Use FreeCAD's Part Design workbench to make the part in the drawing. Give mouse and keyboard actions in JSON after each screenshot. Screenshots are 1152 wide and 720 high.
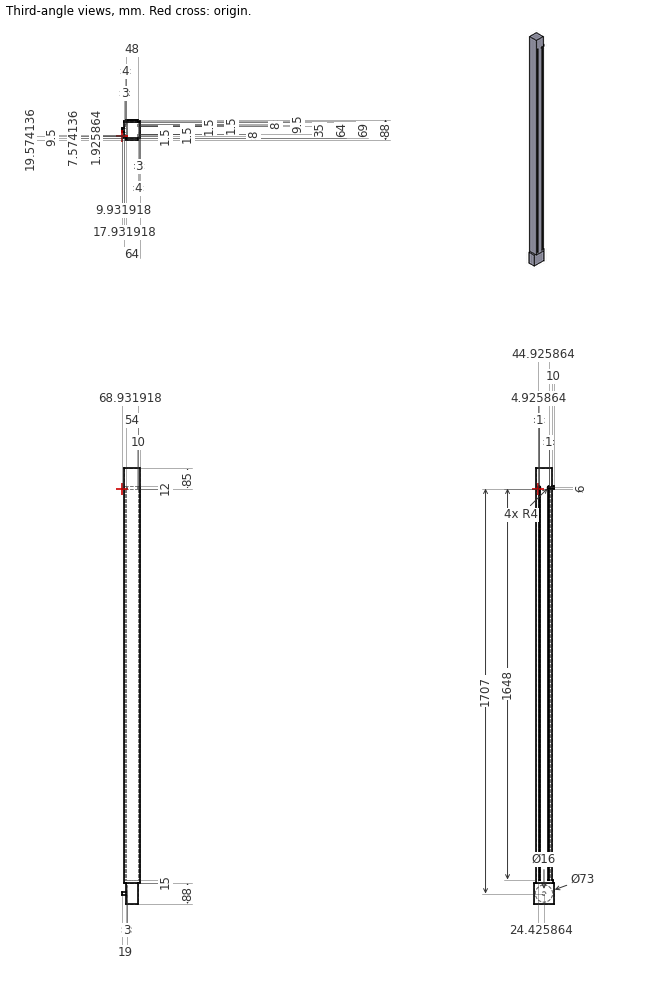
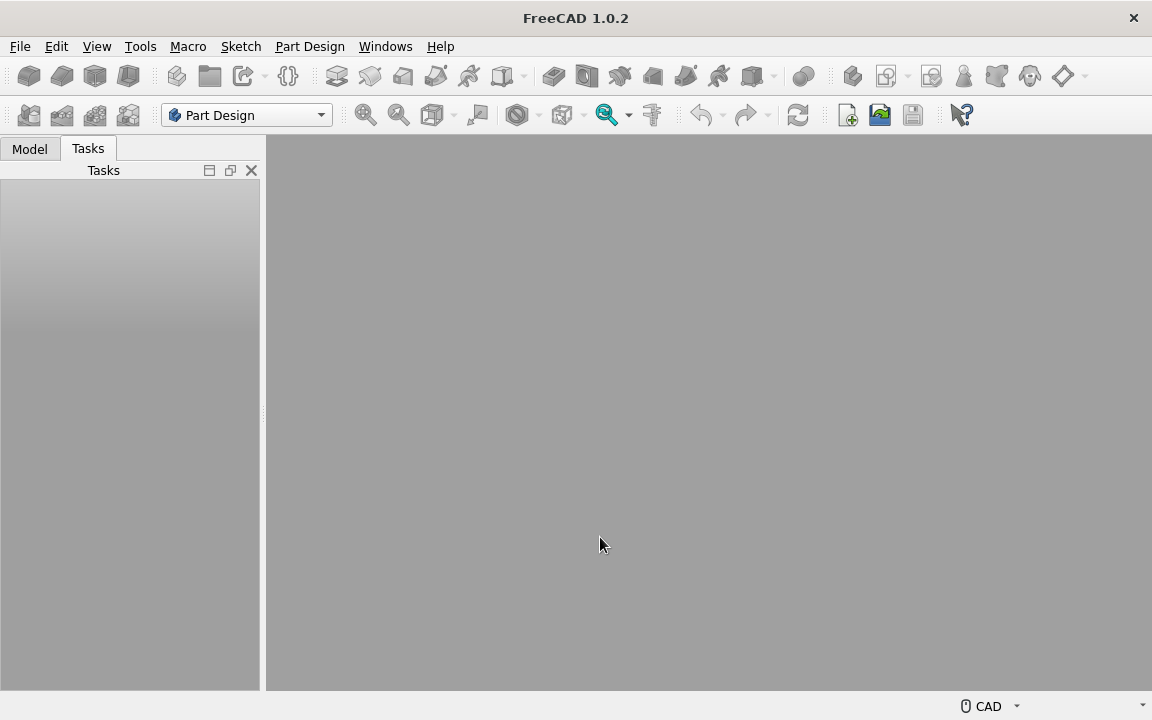
{"action": "left_click", "coordinate": [847, 116]}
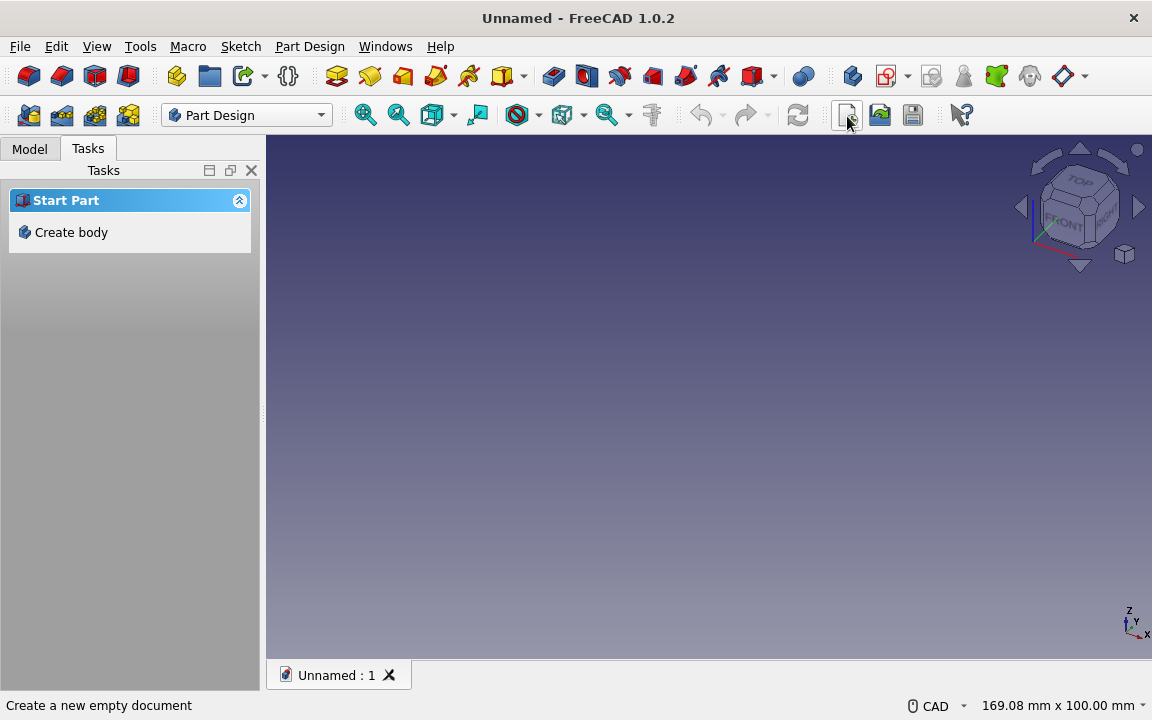
{"action": "left_click", "coordinate": [886, 76]}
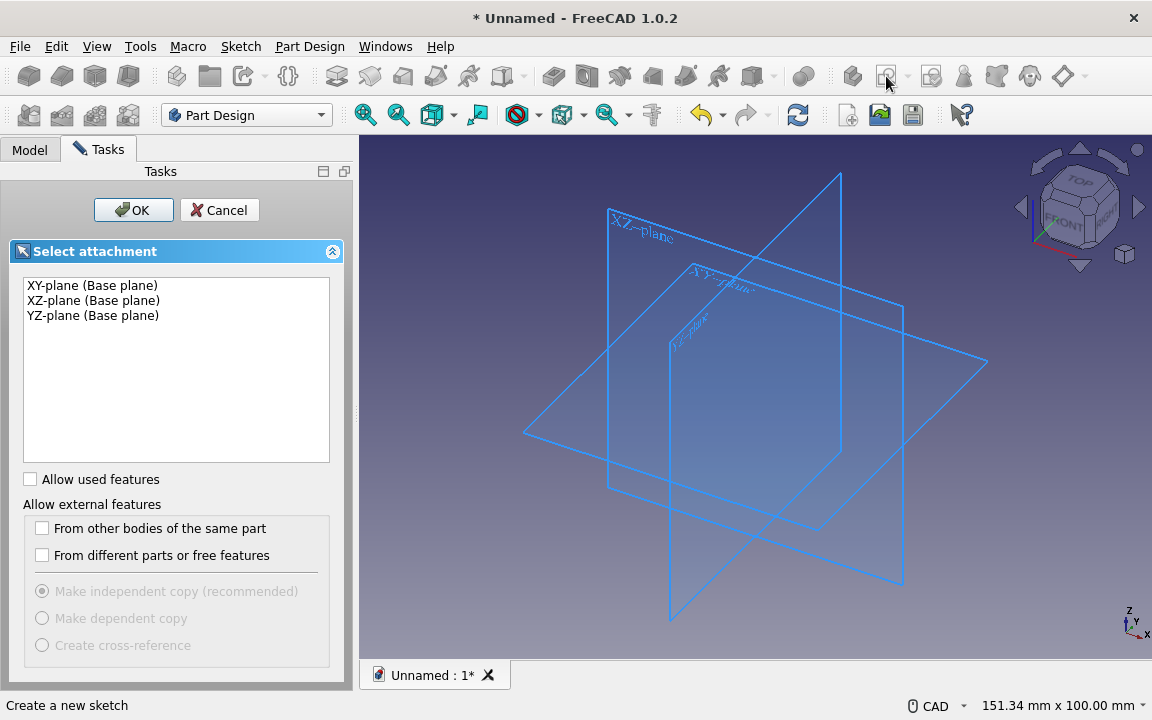
{"action": "left_click", "coordinate": [84, 286]}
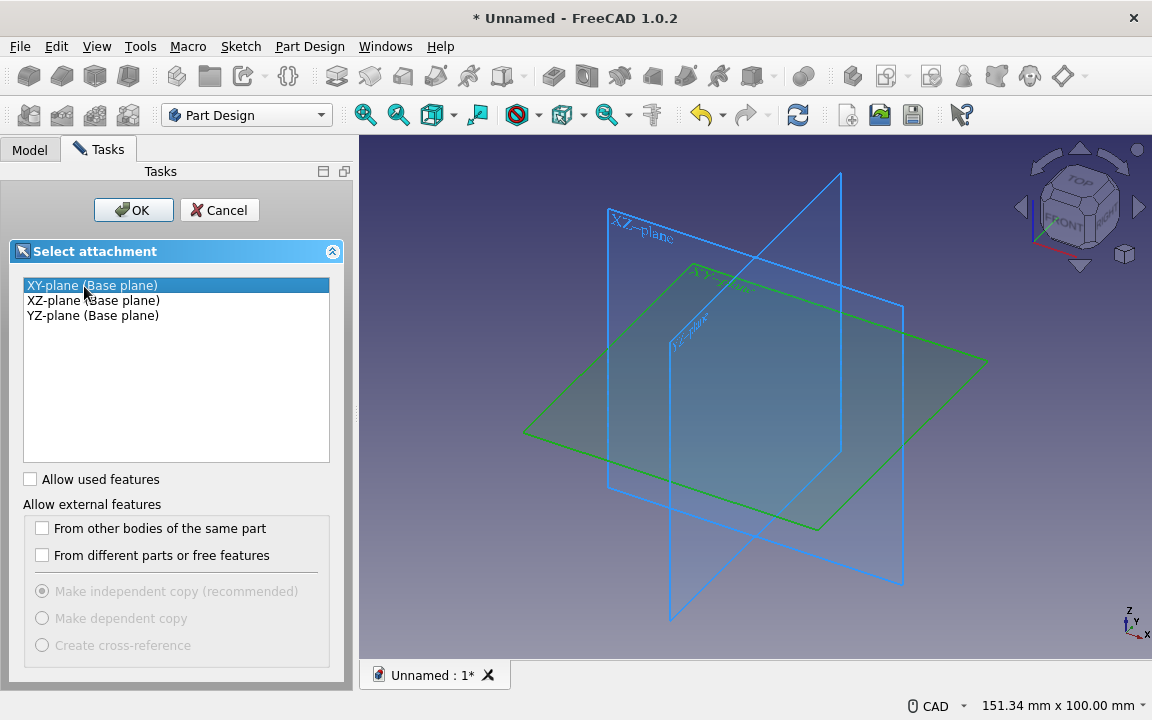
{"action": "left_click", "coordinate": [134, 210]}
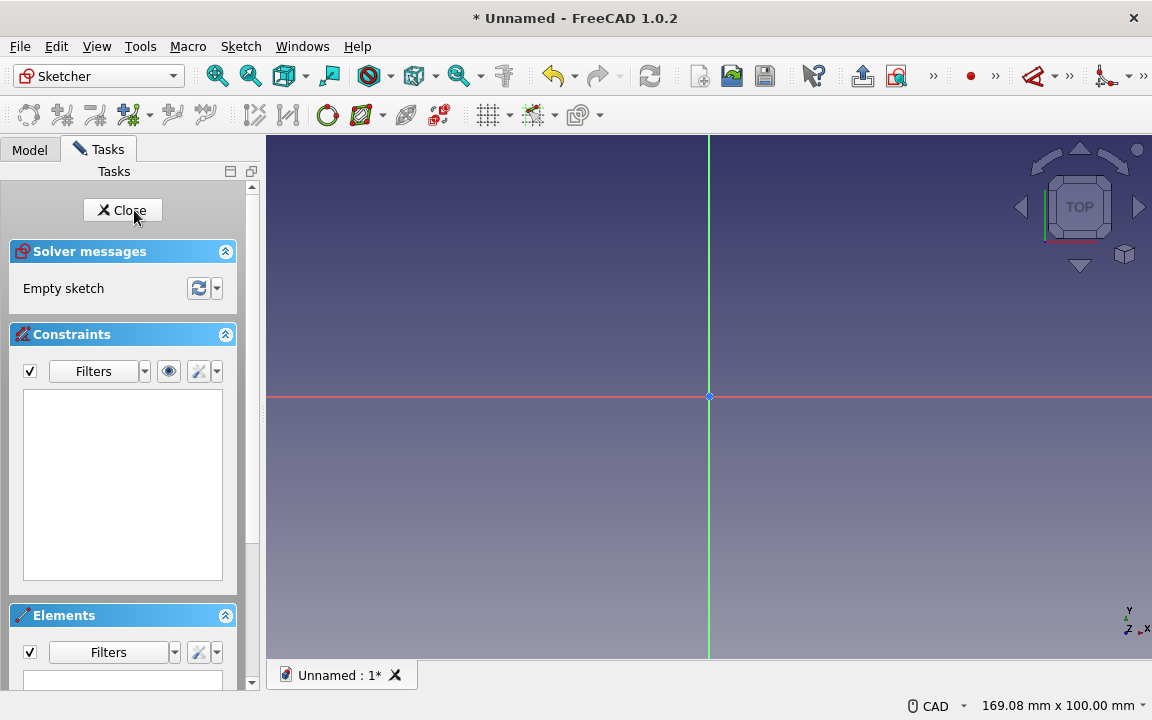
{"action": "scroll", "coordinate": [294, 631], "scroll_direction": "down", "scroll_amount": 1}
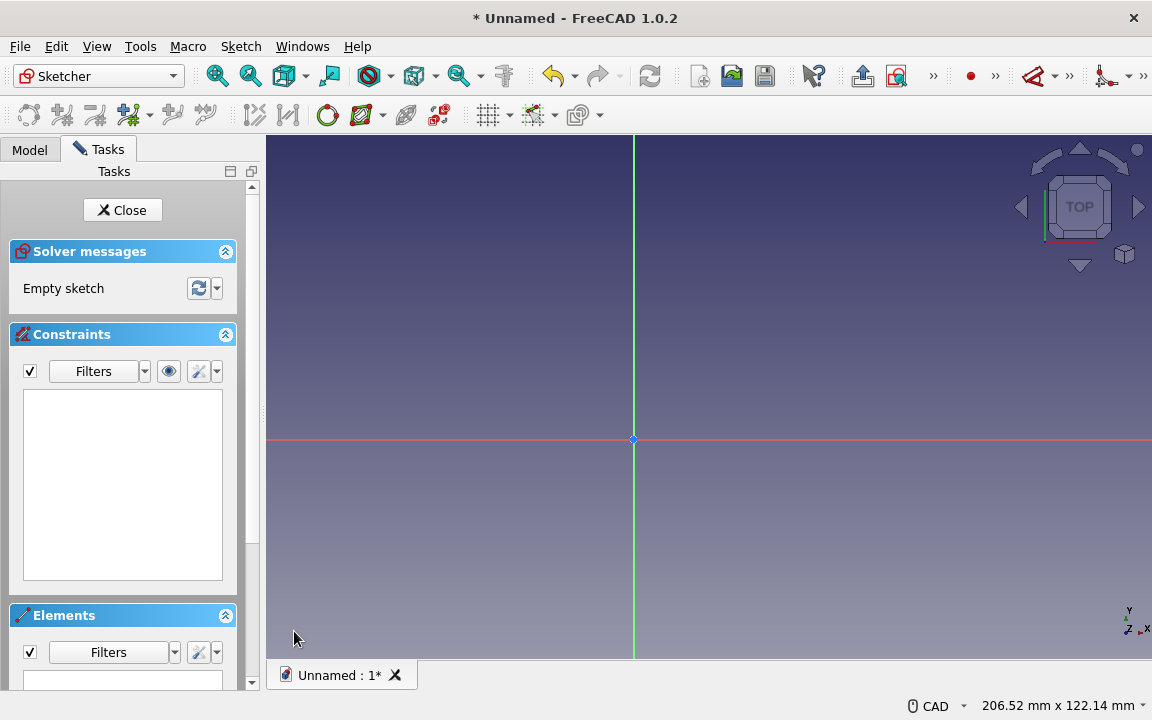
{"action": "key", "text": "g m"}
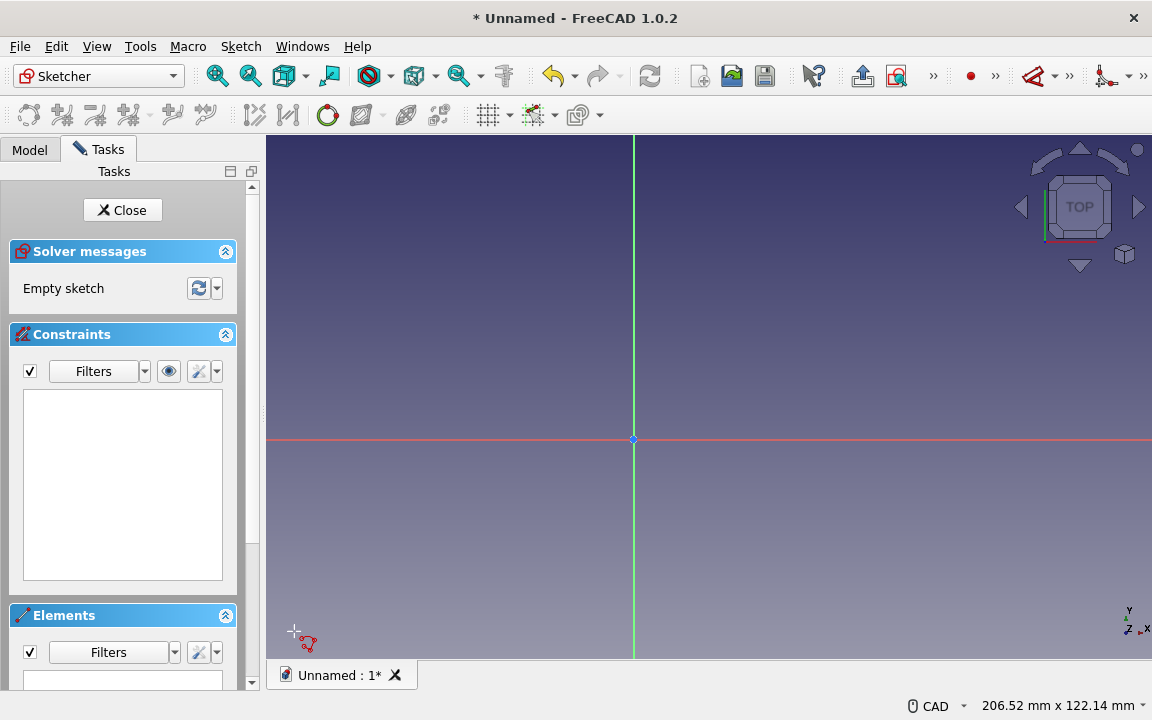
{"action": "scroll", "coordinate": [676, 431], "scroll_direction": "up", "scroll_amount": 4}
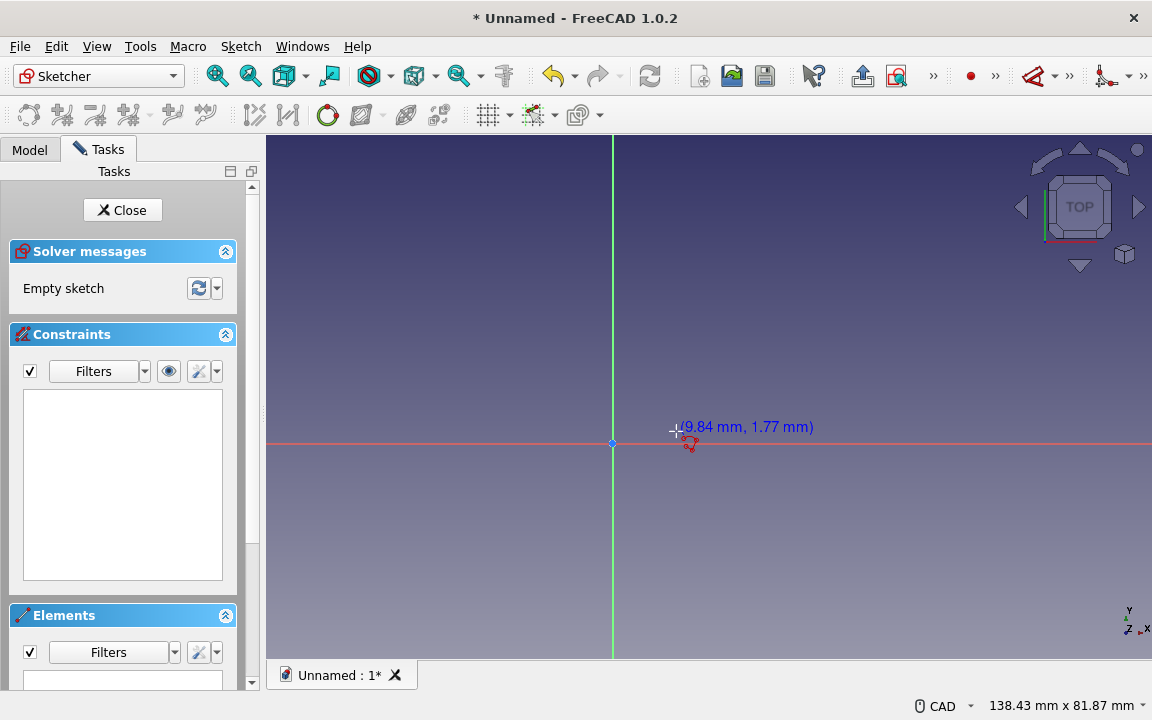
{"action": "left_click", "coordinate": [676, 431]}
{"action": "left_click", "coordinate": [676, 522]}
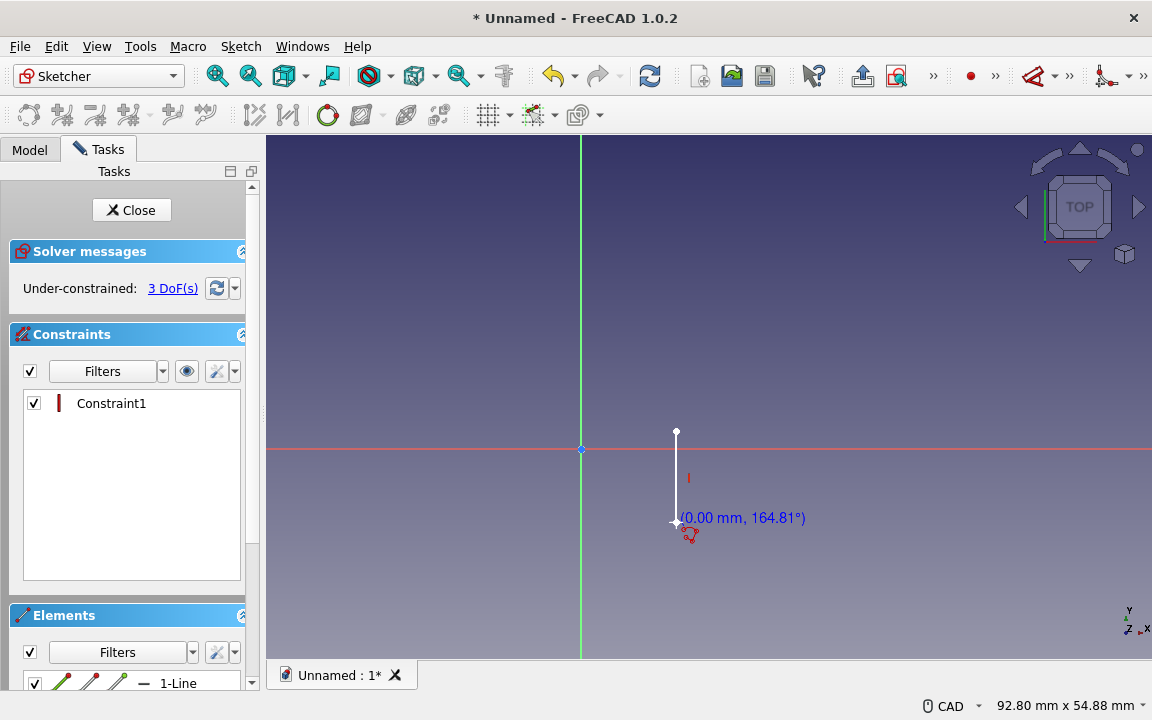
{"action": "scroll", "coordinate": [294, 617], "scroll_direction": "down", "scroll_amount": 3}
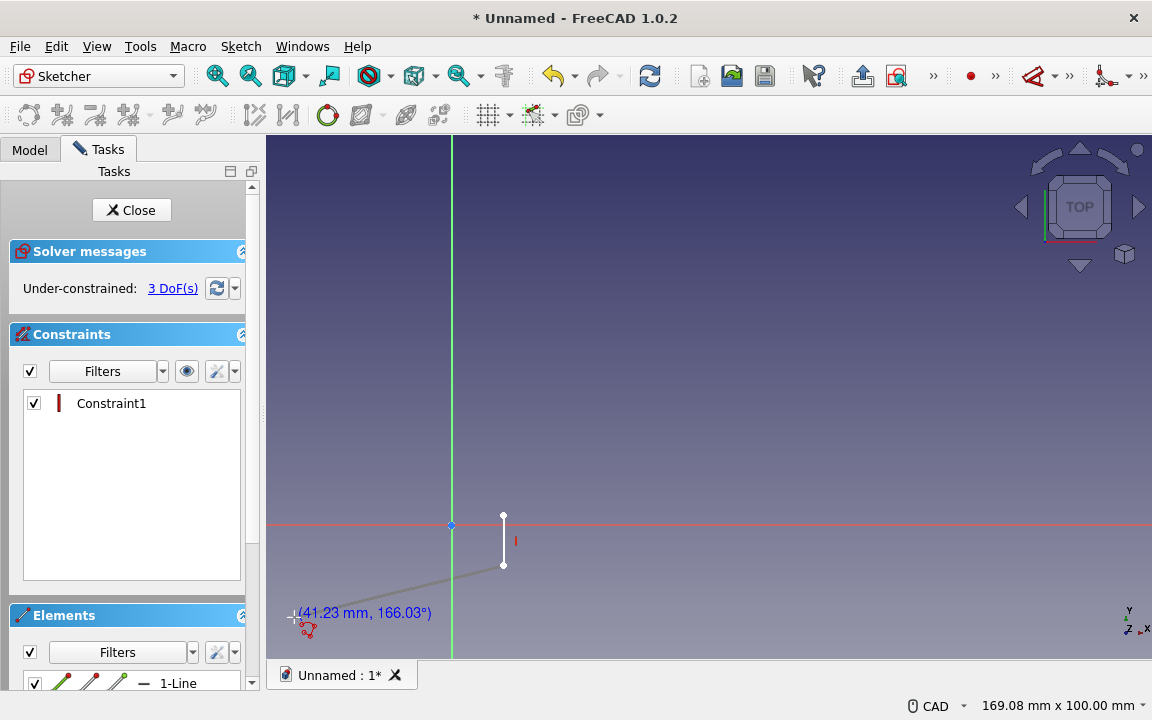
{"action": "left_click", "coordinate": [839, 565]}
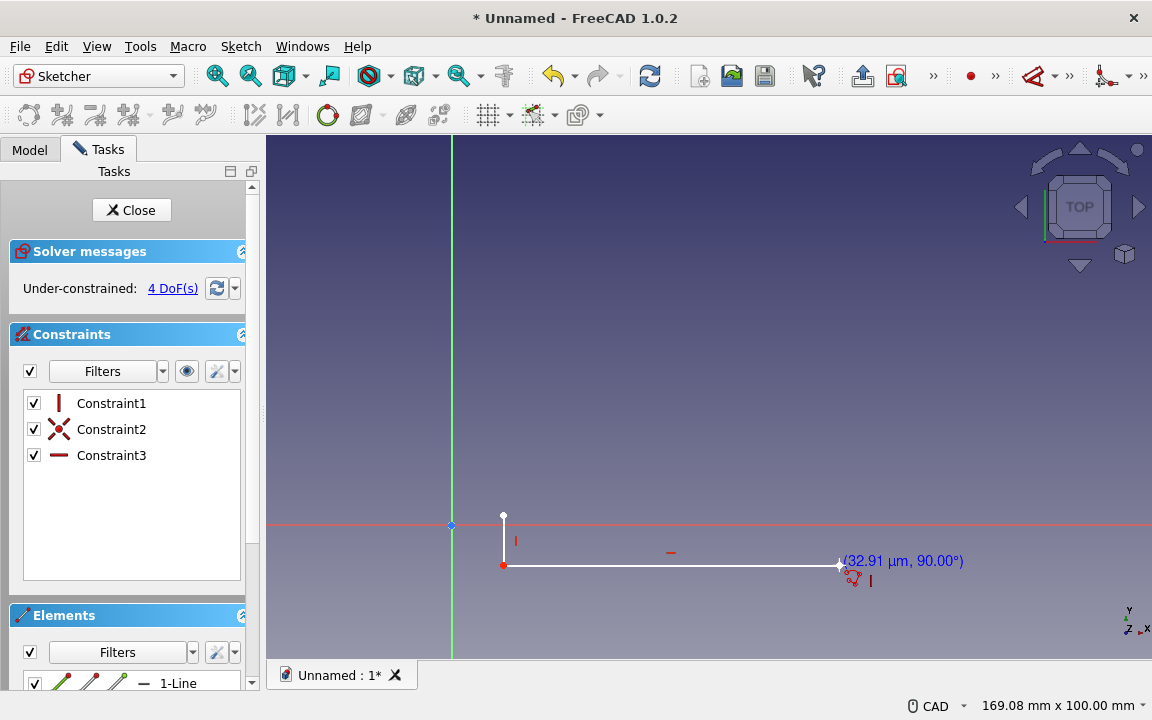
{"action": "scroll", "coordinate": [839, 515], "scroll_direction": "up", "scroll_amount": 3}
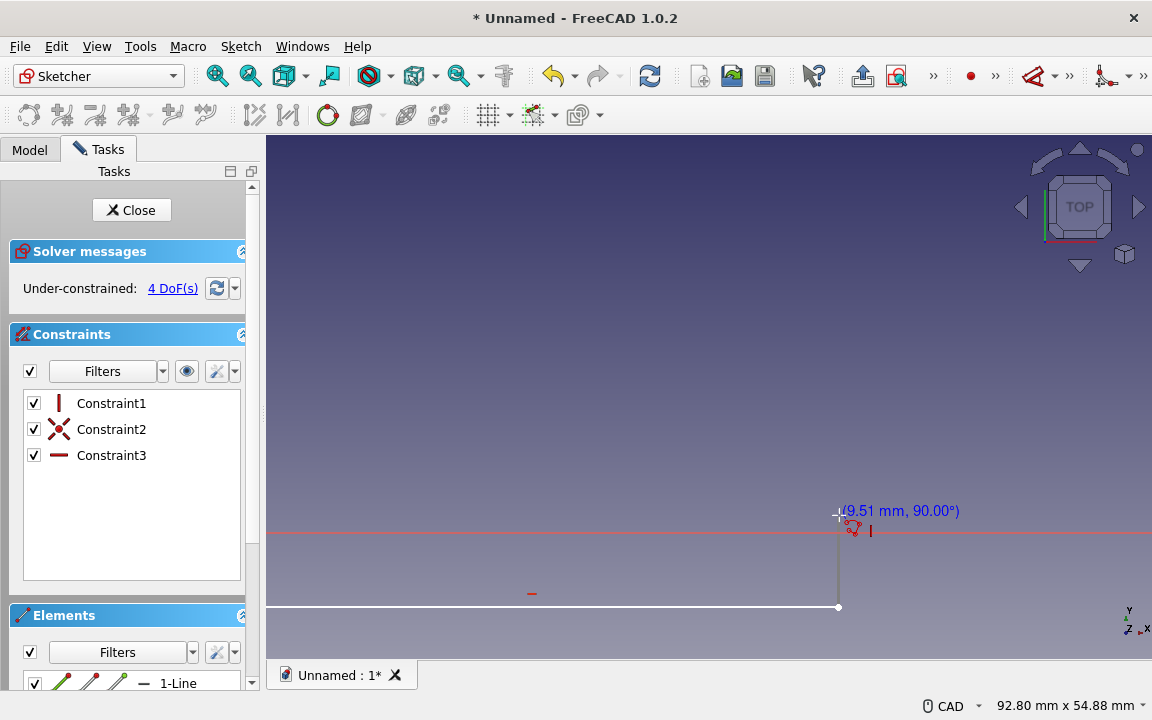
{"action": "left_click", "coordinate": [838, 515]}
{"action": "left_click", "coordinate": [810, 515]}